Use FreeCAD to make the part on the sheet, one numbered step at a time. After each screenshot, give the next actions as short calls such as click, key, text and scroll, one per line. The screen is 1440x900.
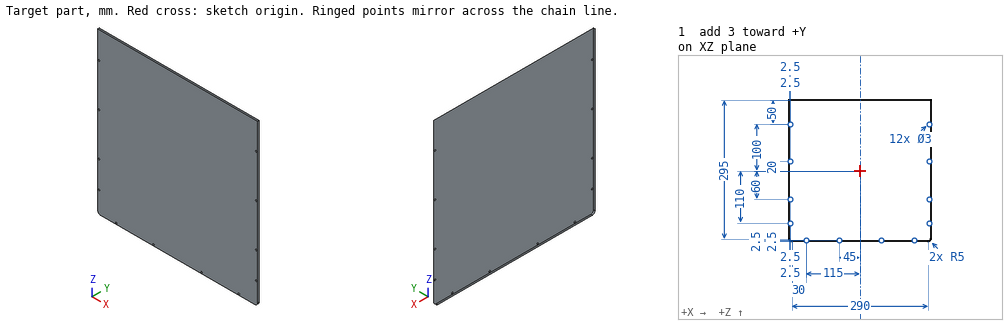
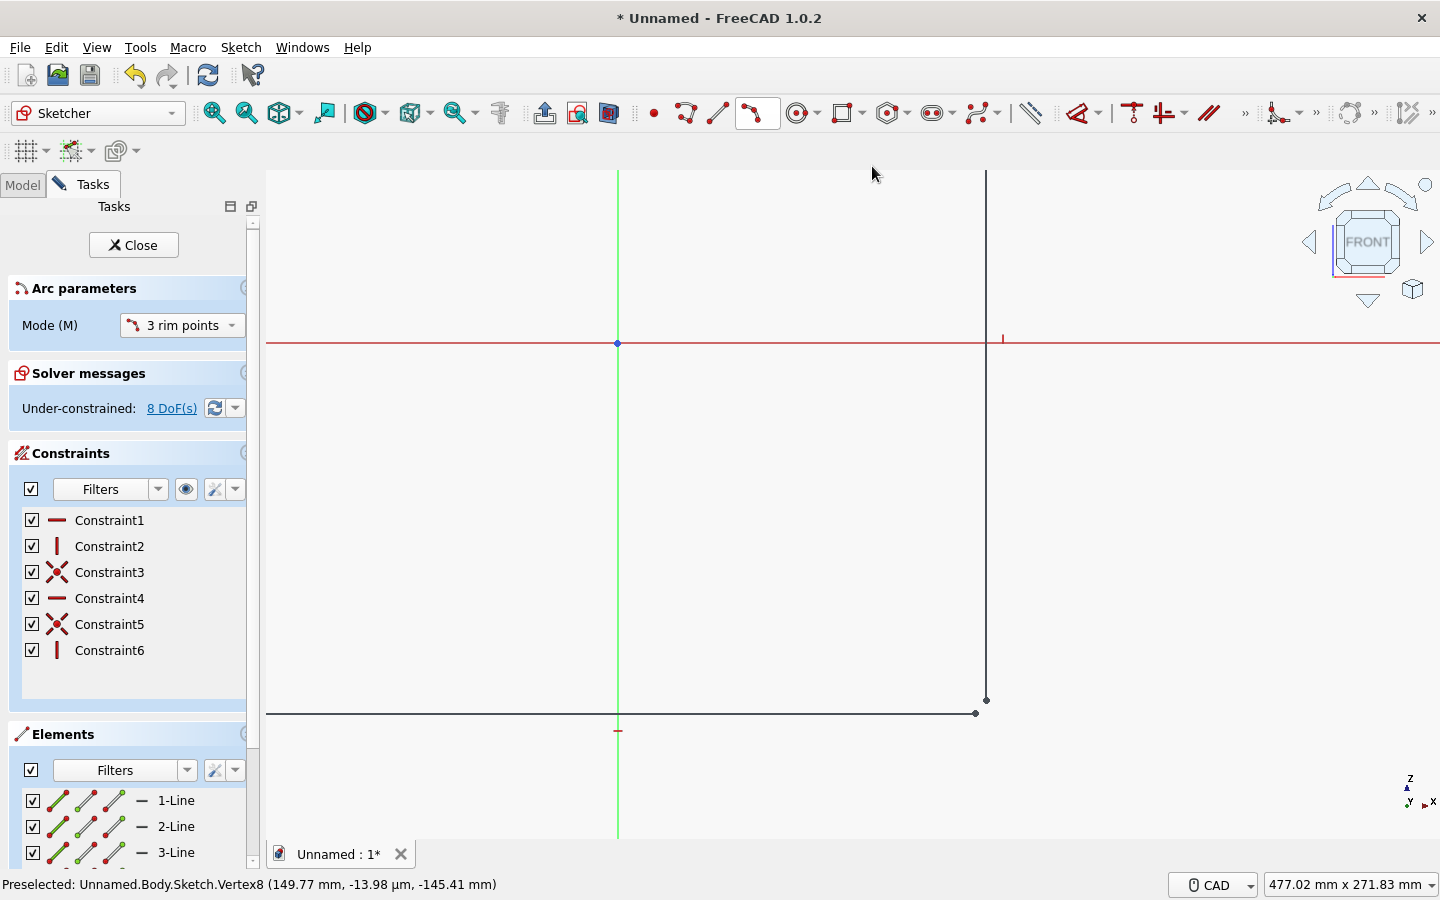
scroll(987, 701, down, 3)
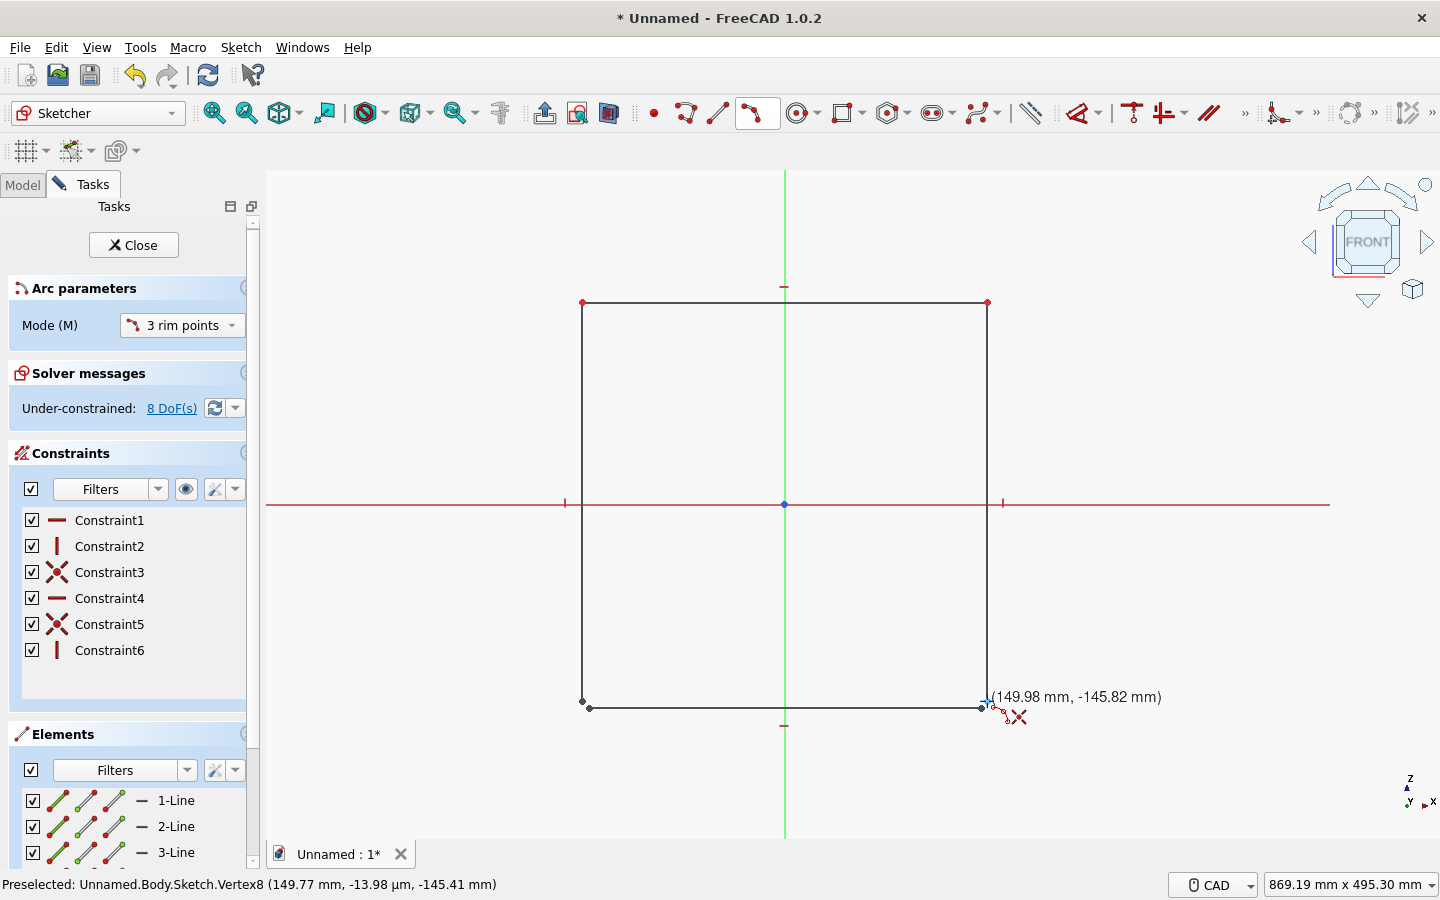
scroll(589, 708, up, 3)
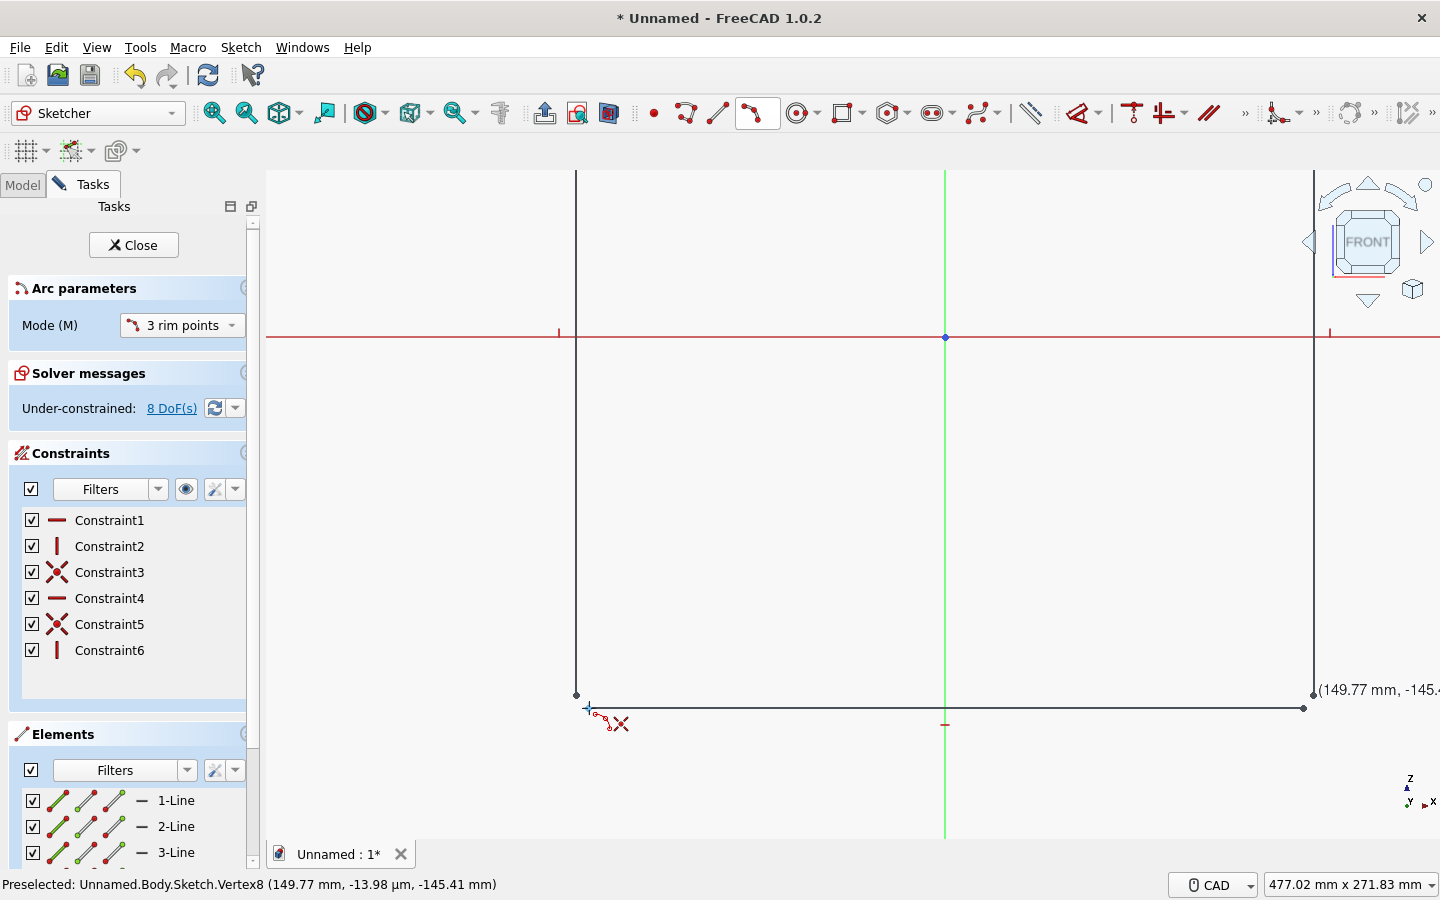
click(589, 708)
click(576, 695)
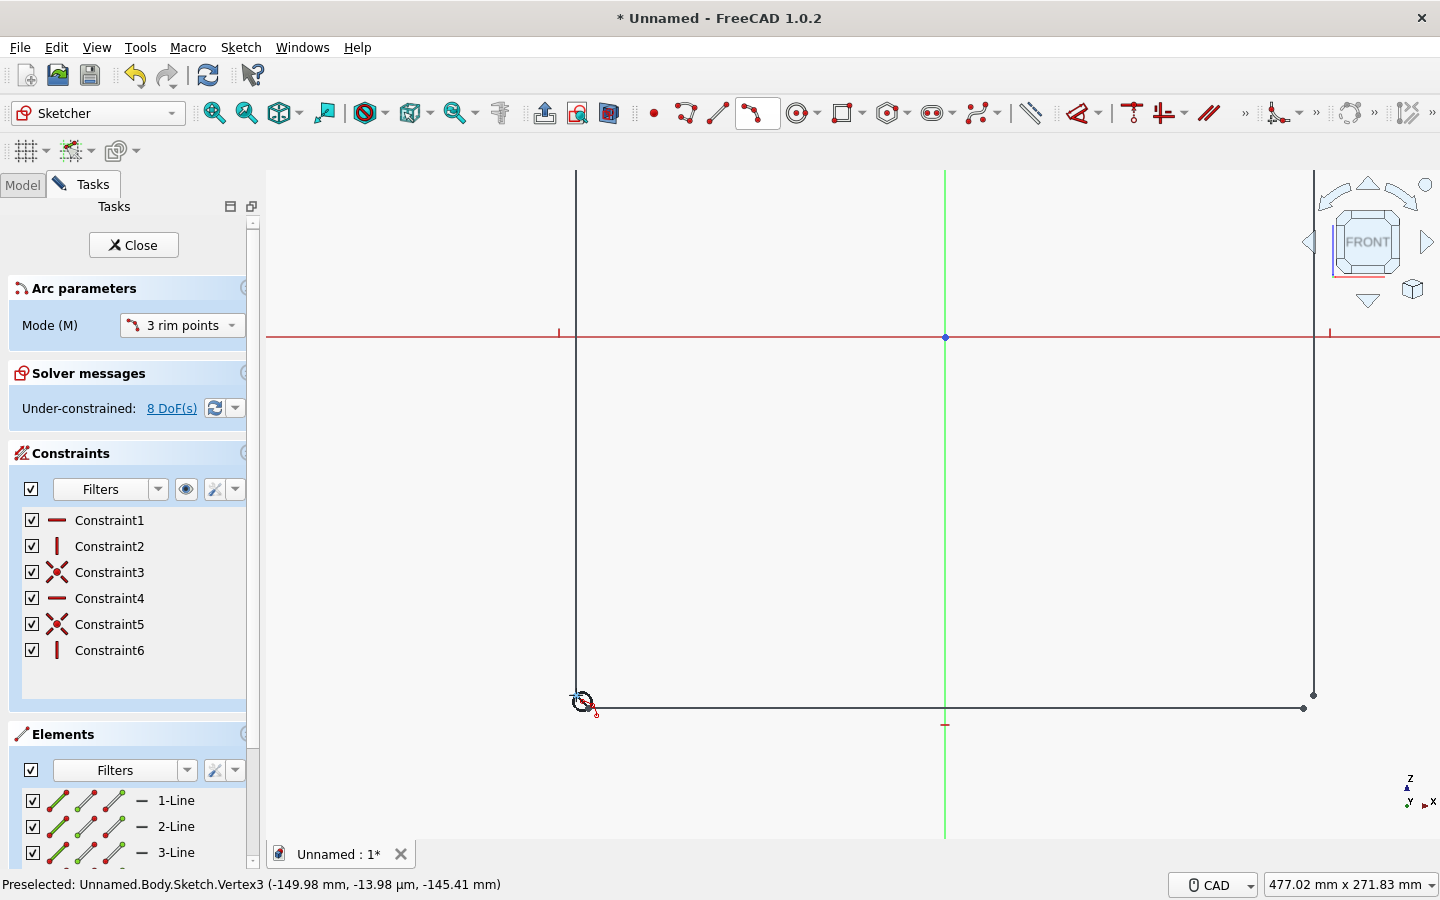
scroll(580, 703, up, 8)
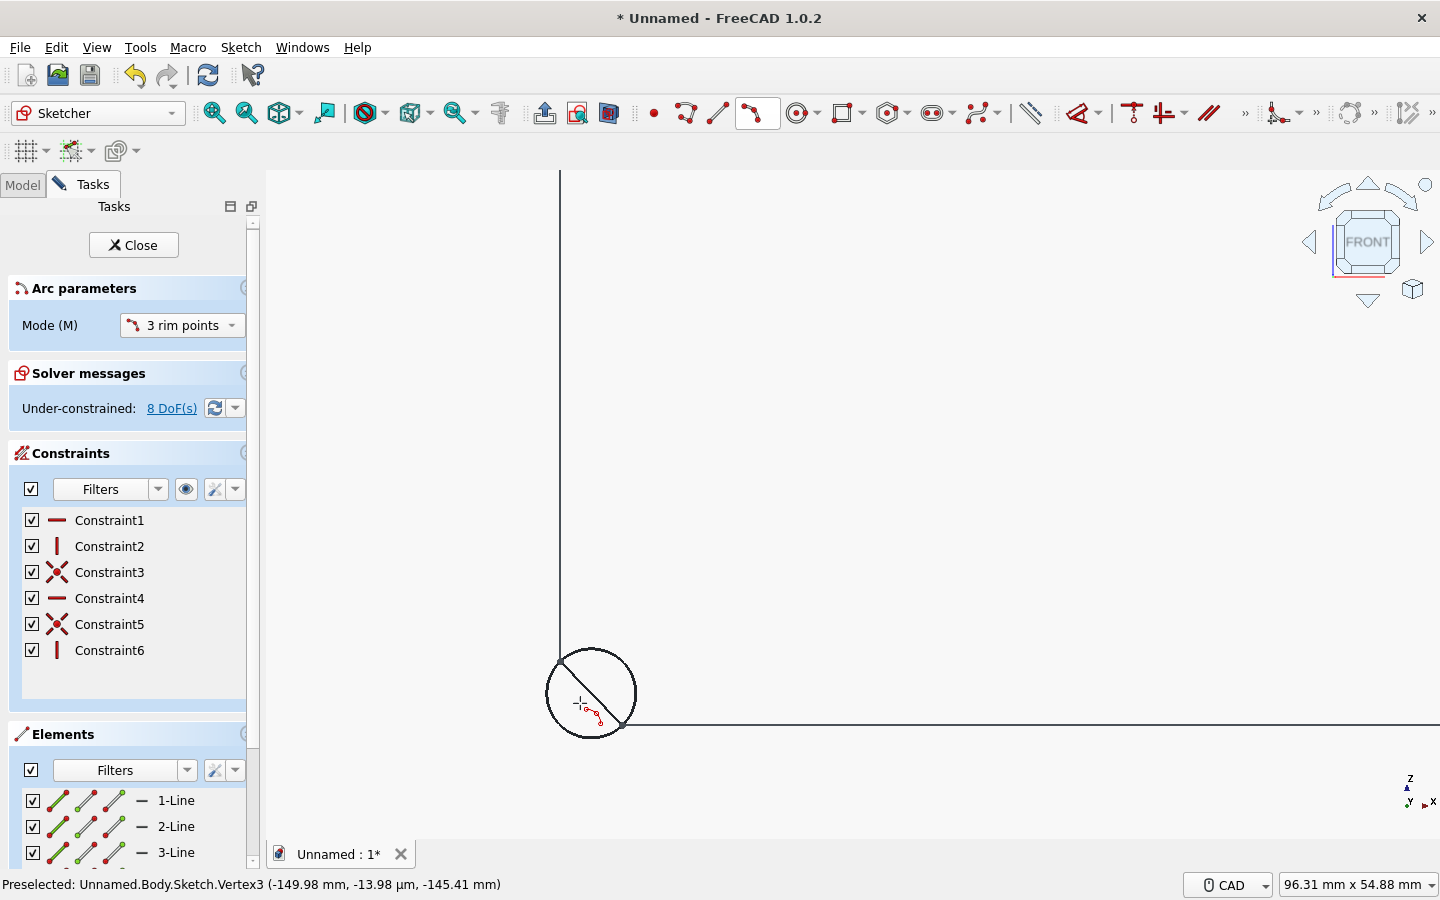
click(578, 699)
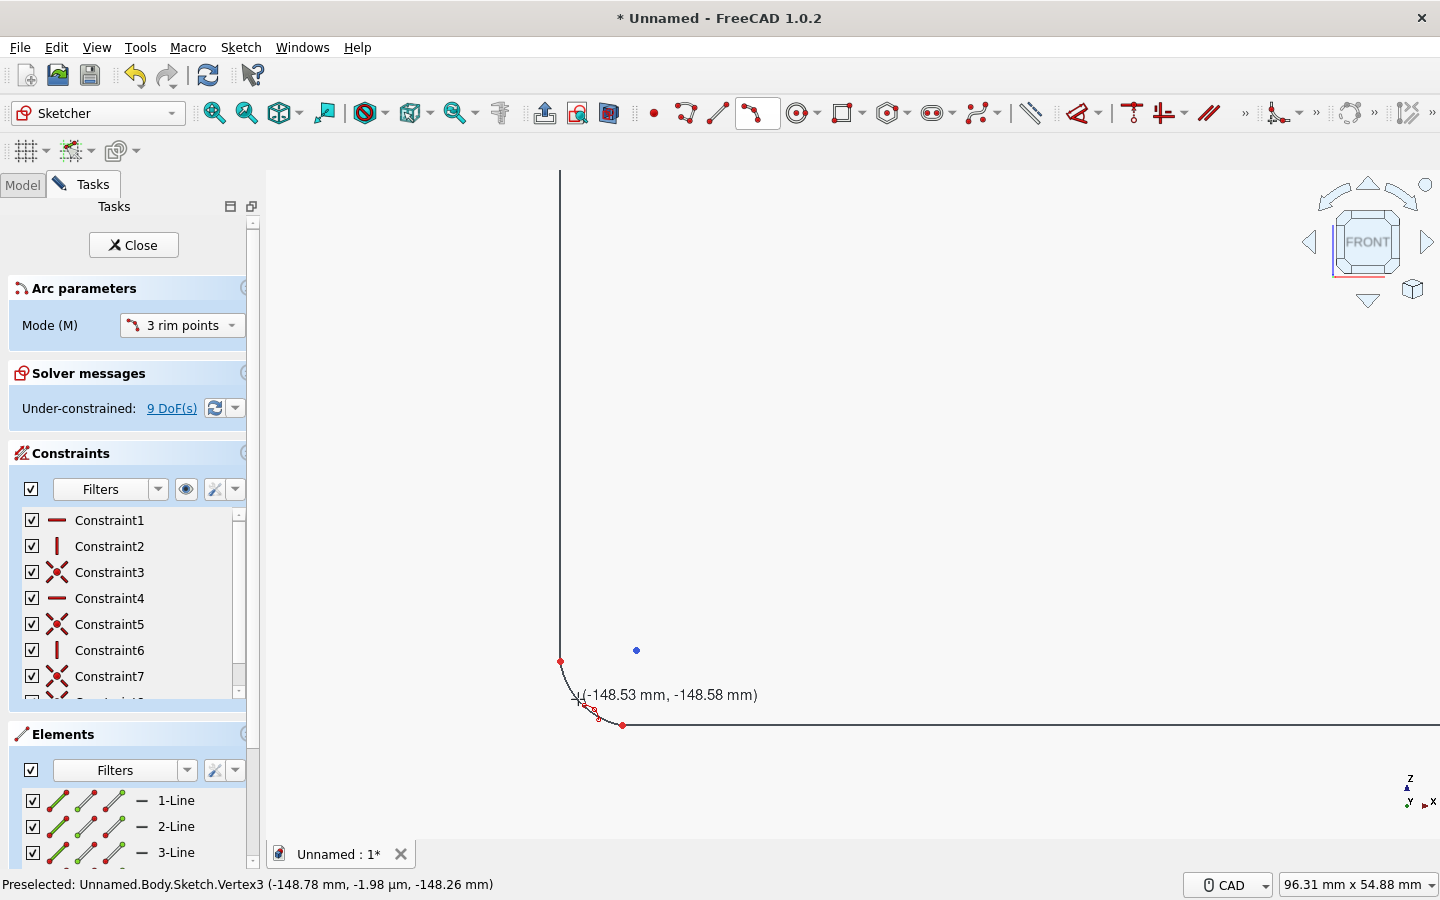
scroll(585, 706, down, 11)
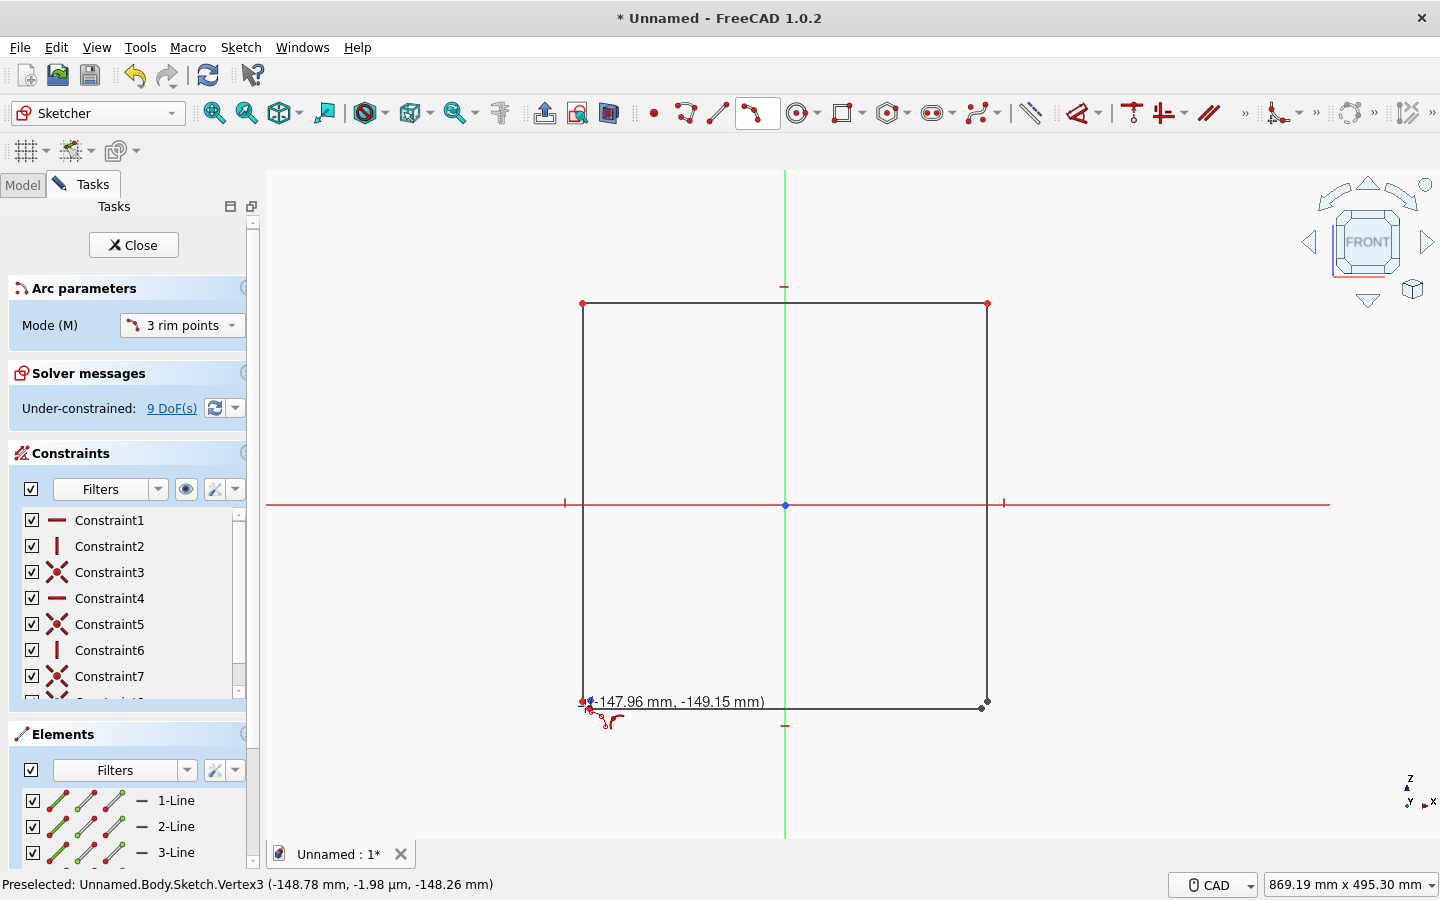
scroll(988, 701, up, 3)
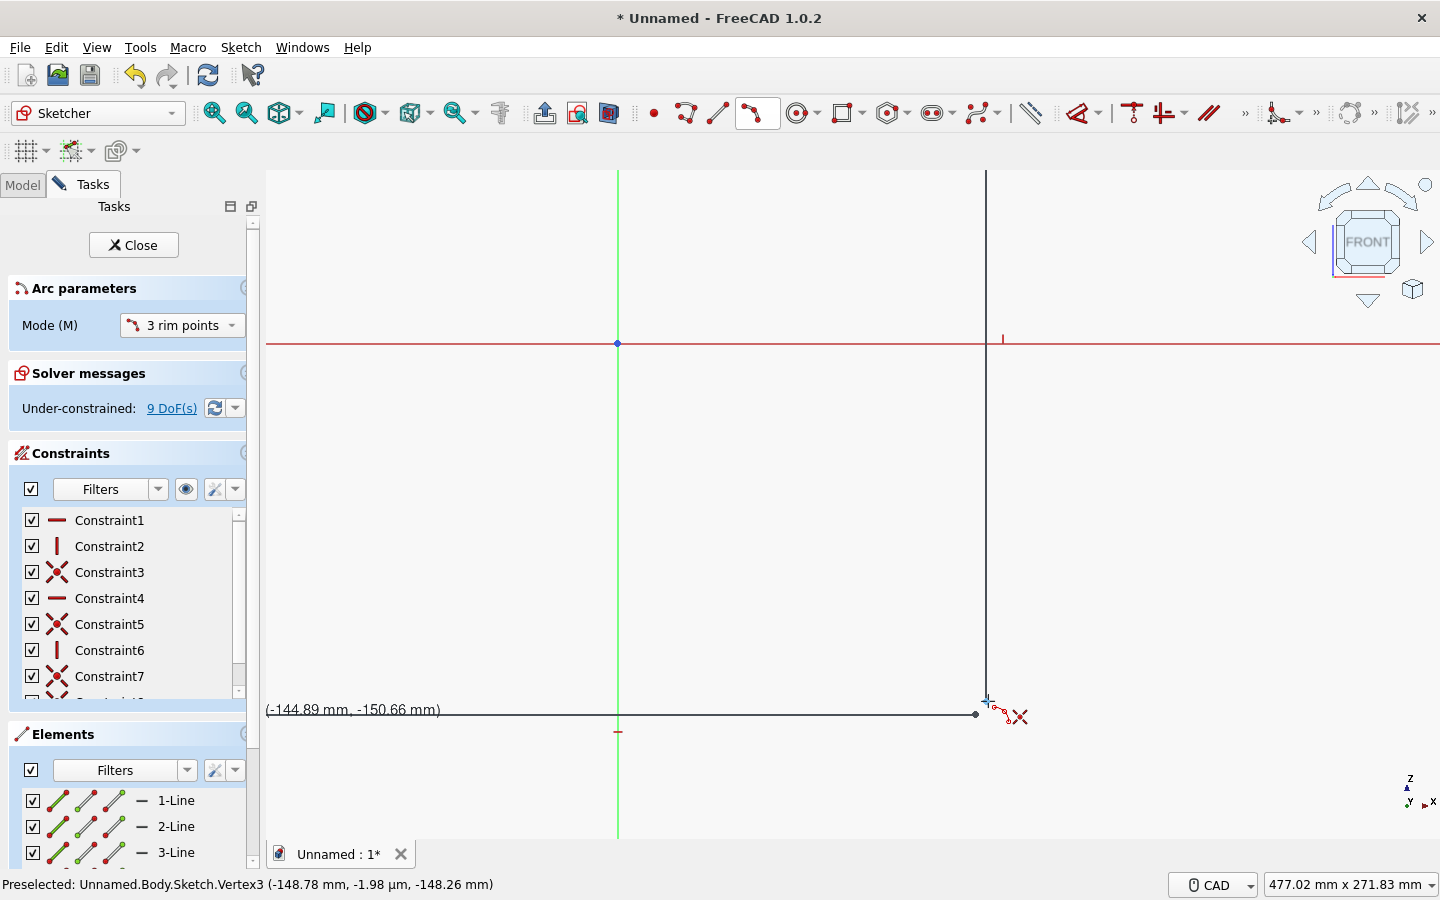
click(986, 702)
click(975, 715)